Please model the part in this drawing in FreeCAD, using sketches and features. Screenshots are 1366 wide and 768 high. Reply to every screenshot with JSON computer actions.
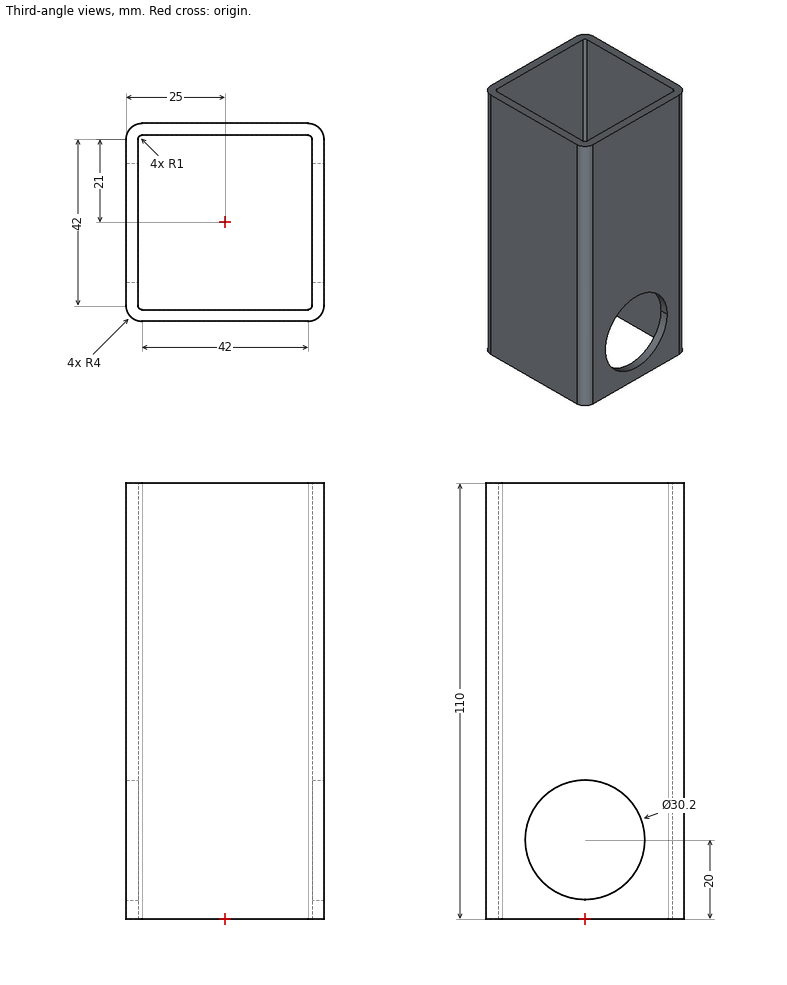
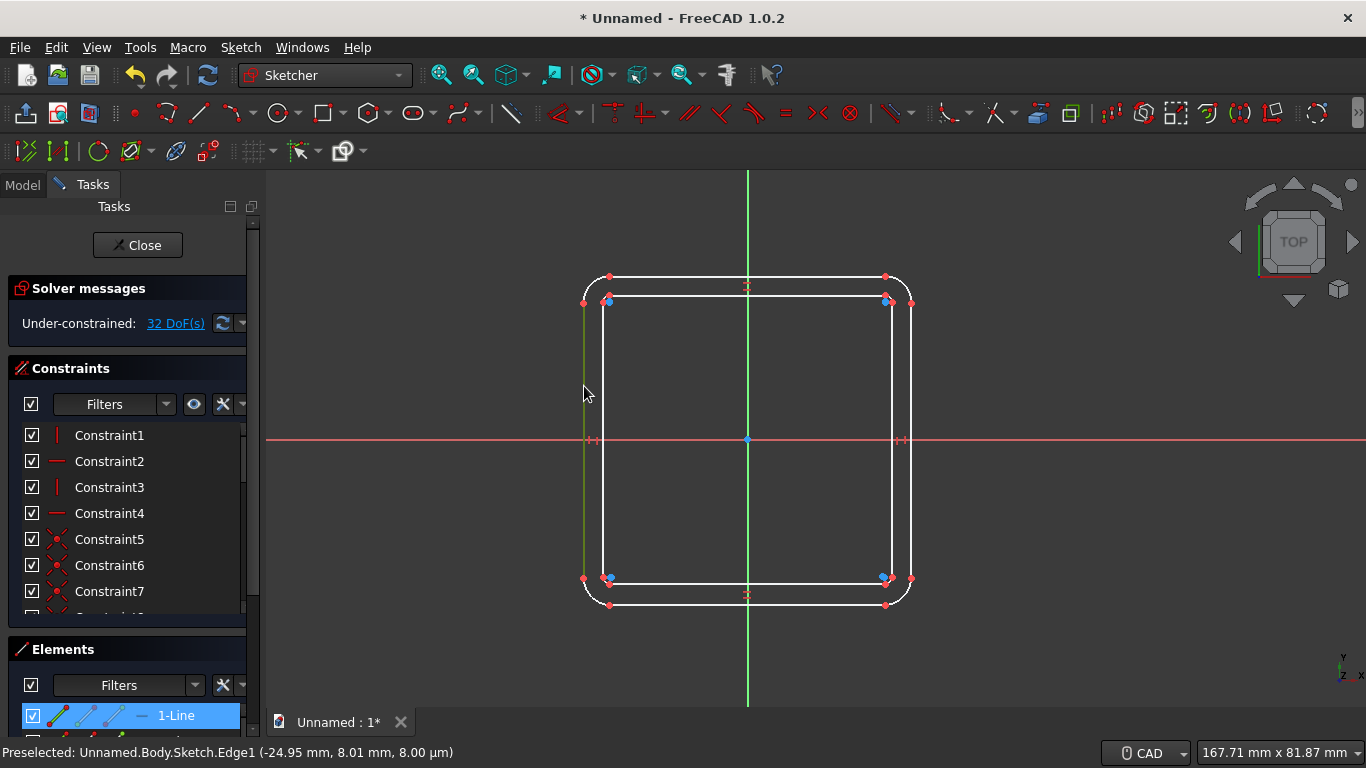
{"action": "left_click", "coordinate": [587, 590]}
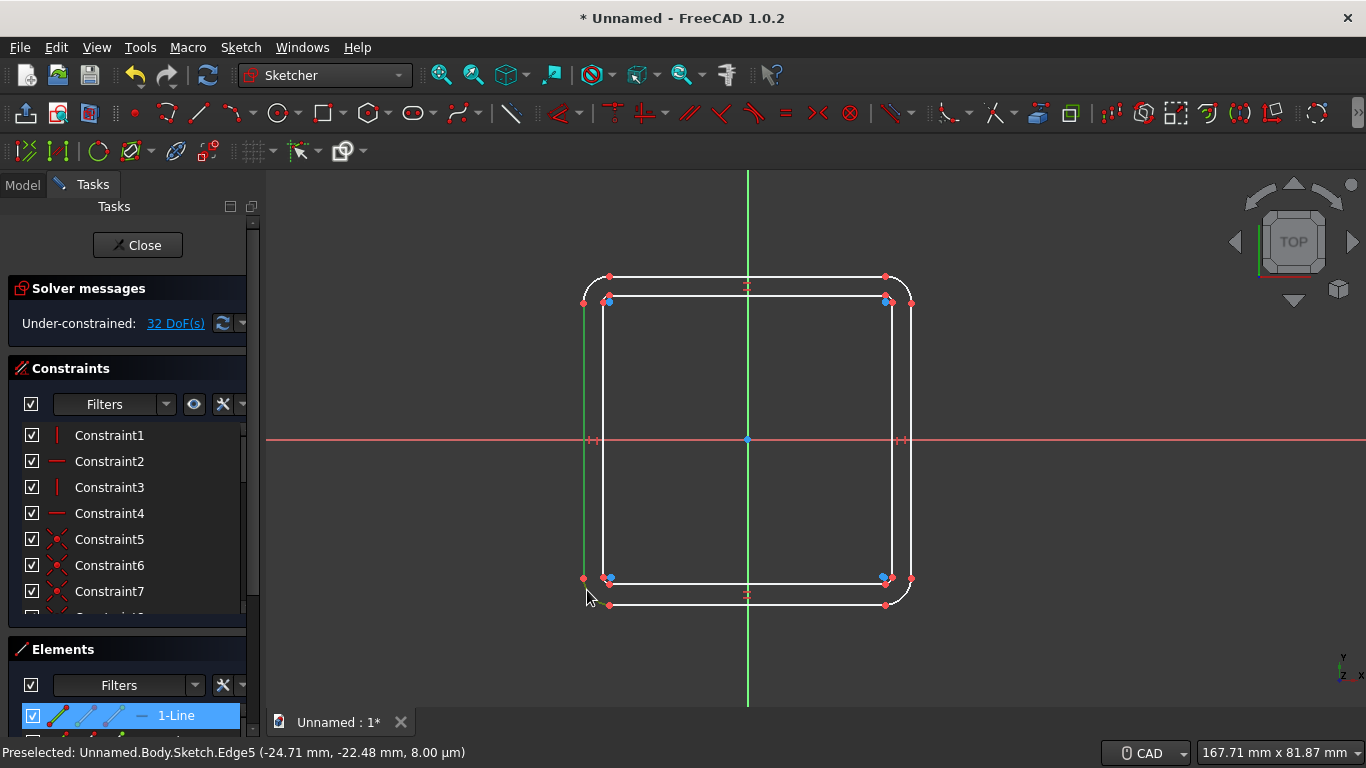
{"action": "left_click", "coordinate": [754, 114]}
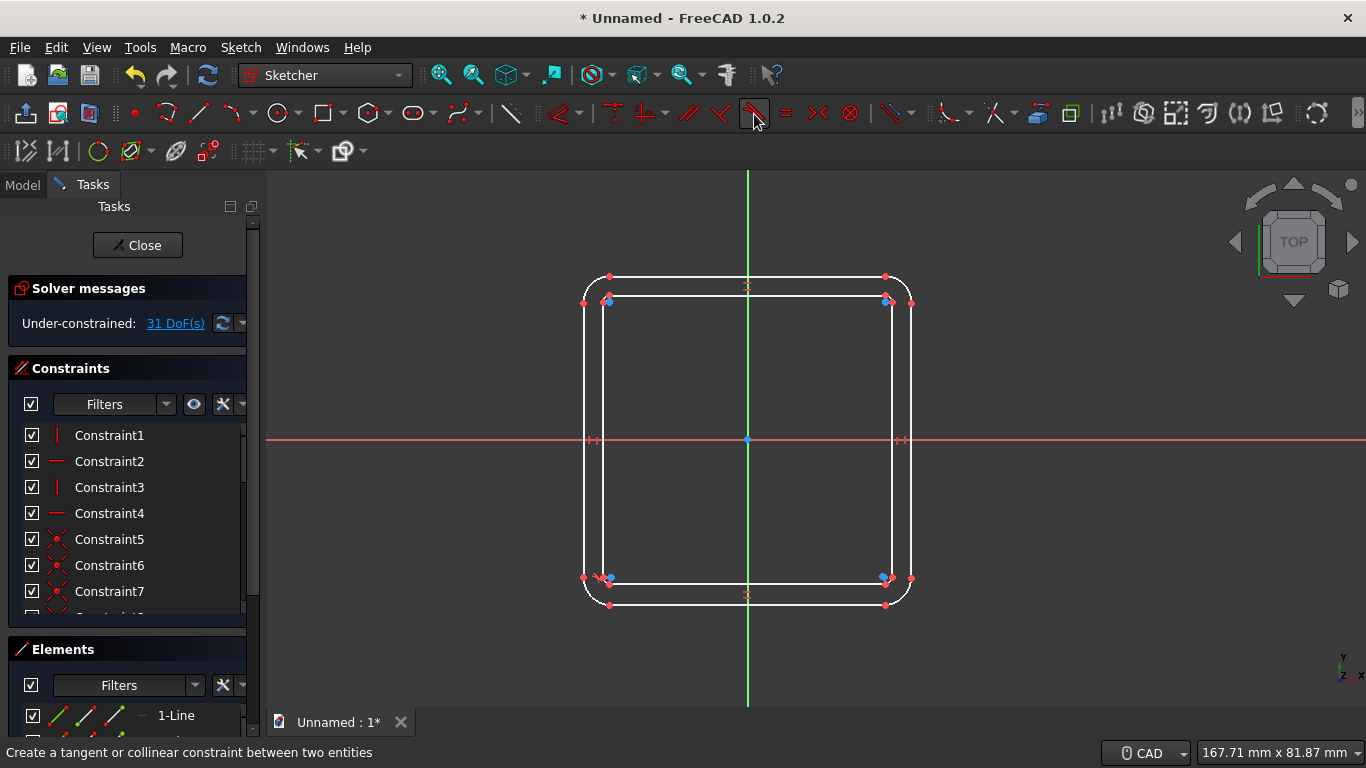
{"action": "left_click", "coordinate": [584, 386]}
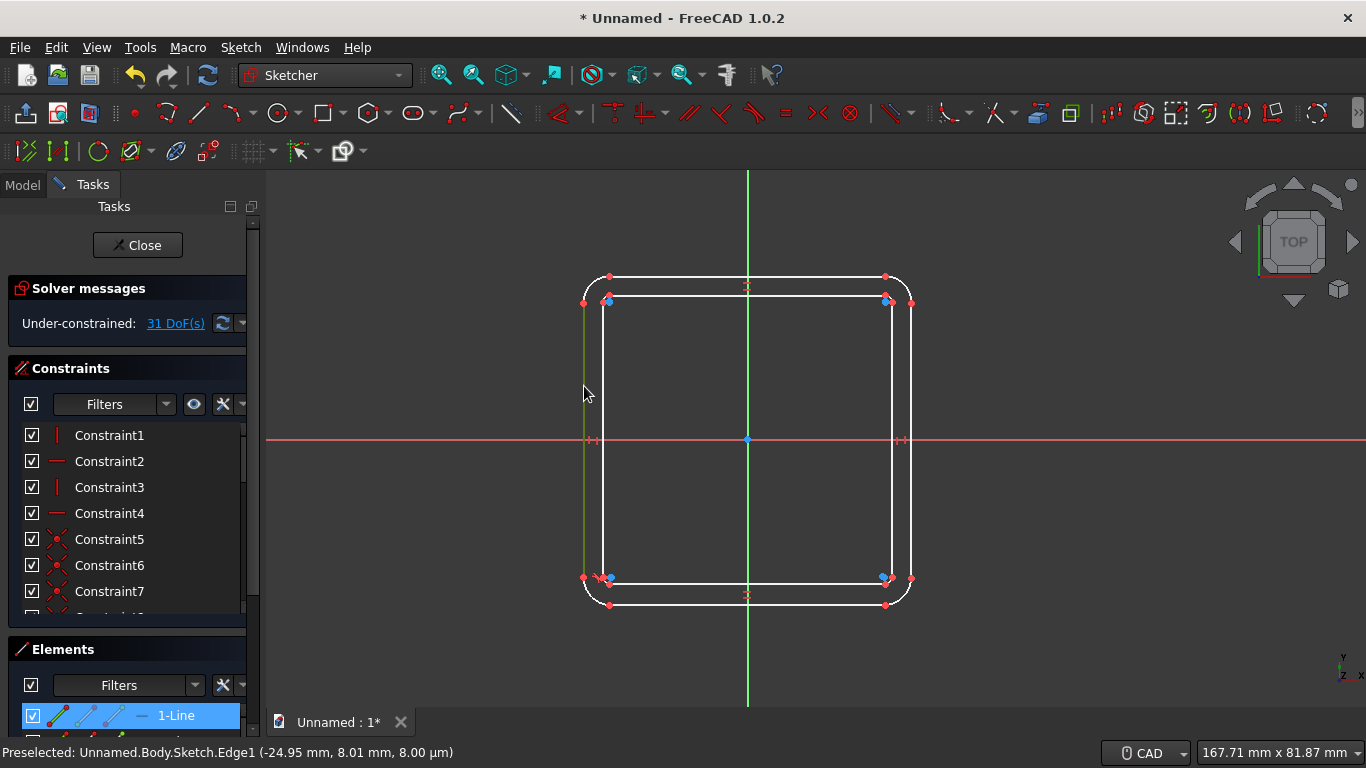
{"action": "left_click", "coordinate": [598, 279]}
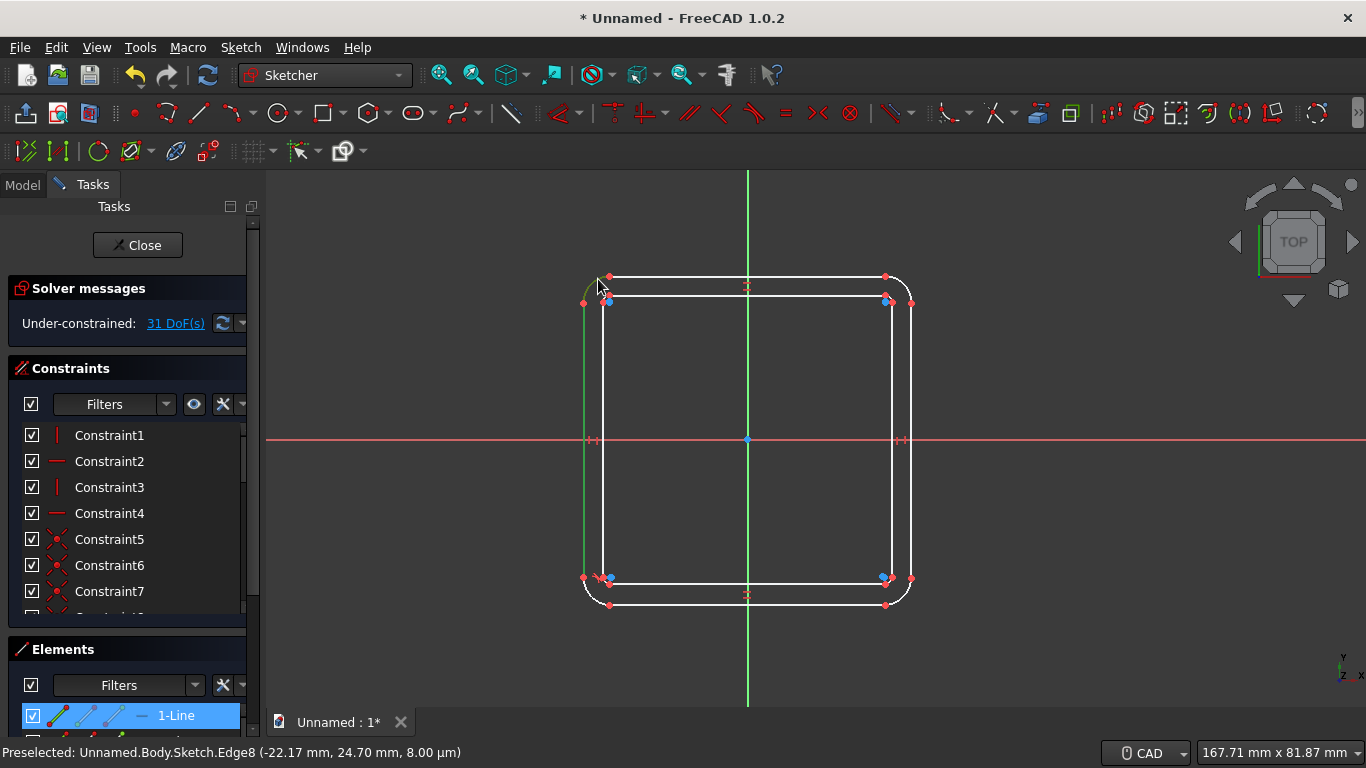
{"action": "left_click", "coordinate": [754, 114]}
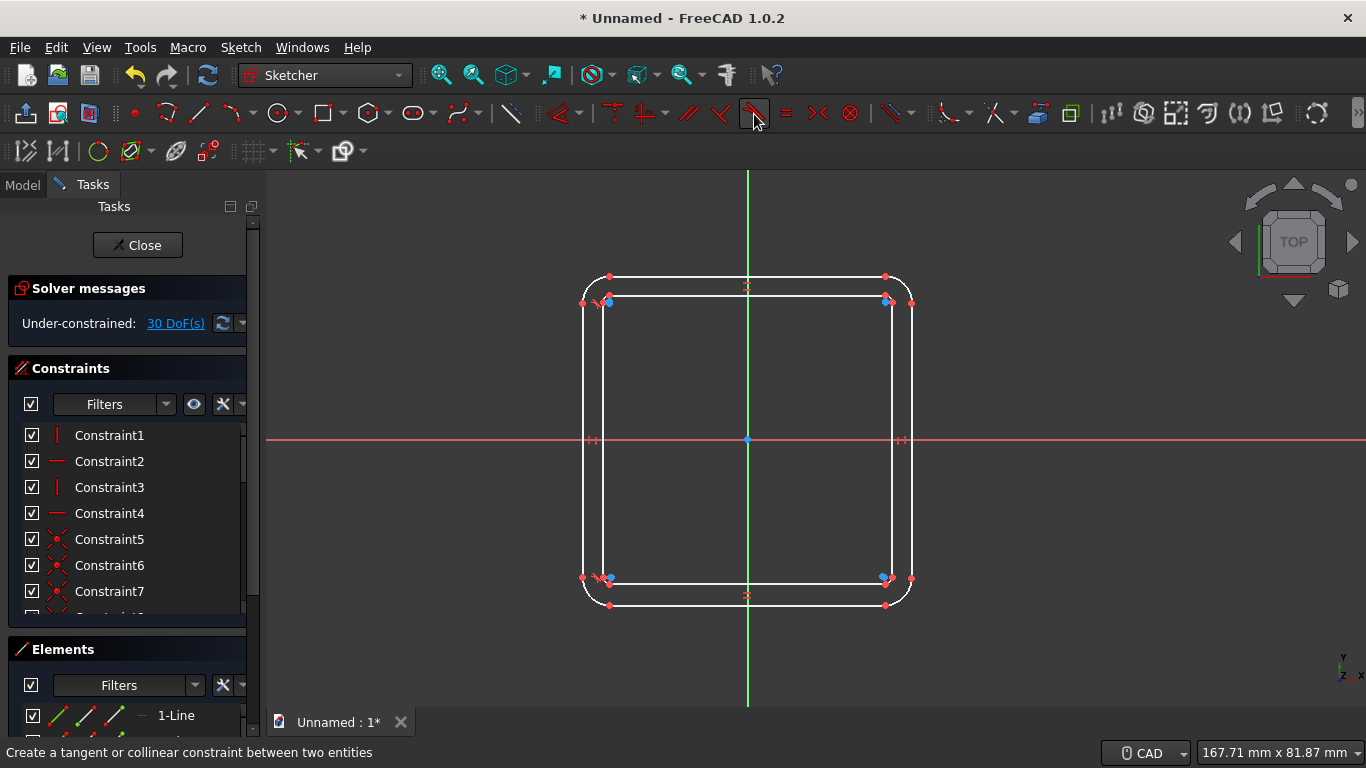
{"action": "left_click", "coordinate": [692, 606]}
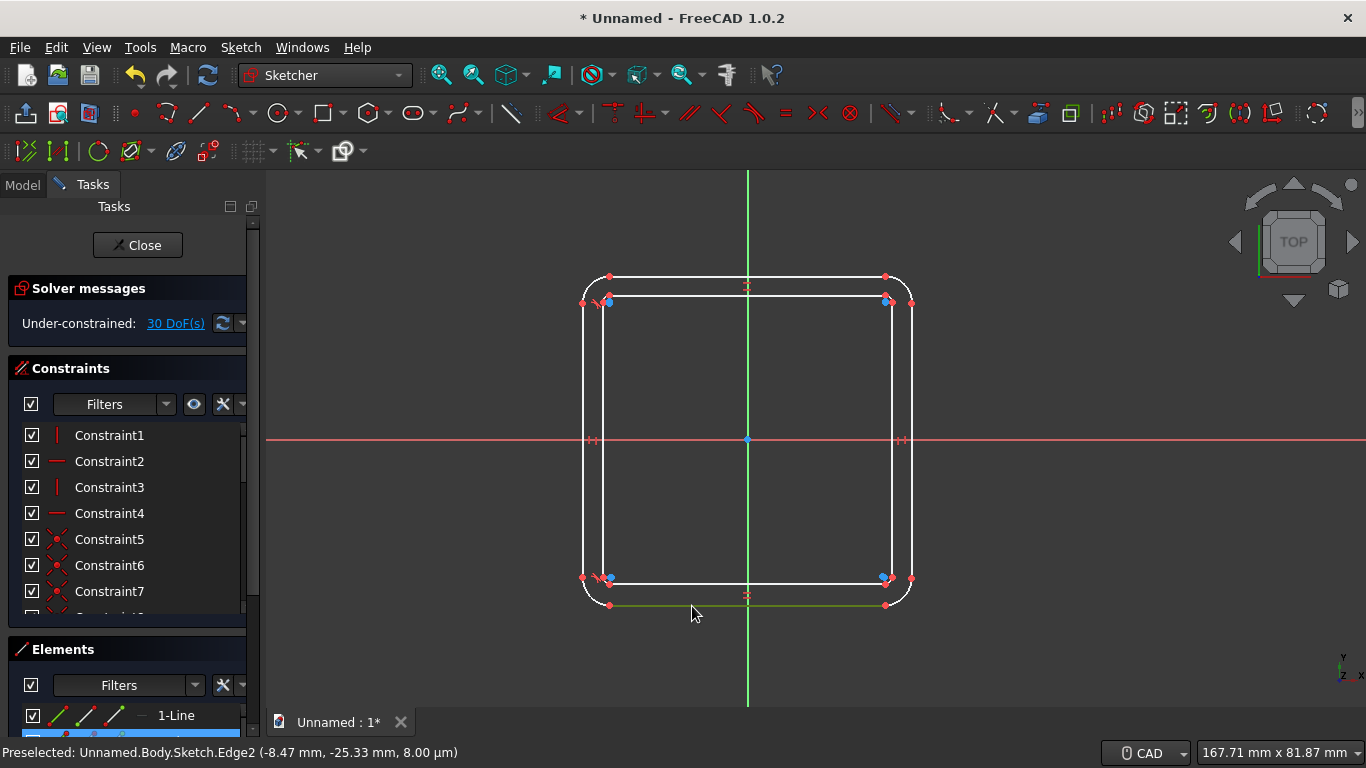
{"action": "left_click", "coordinate": [586, 590]}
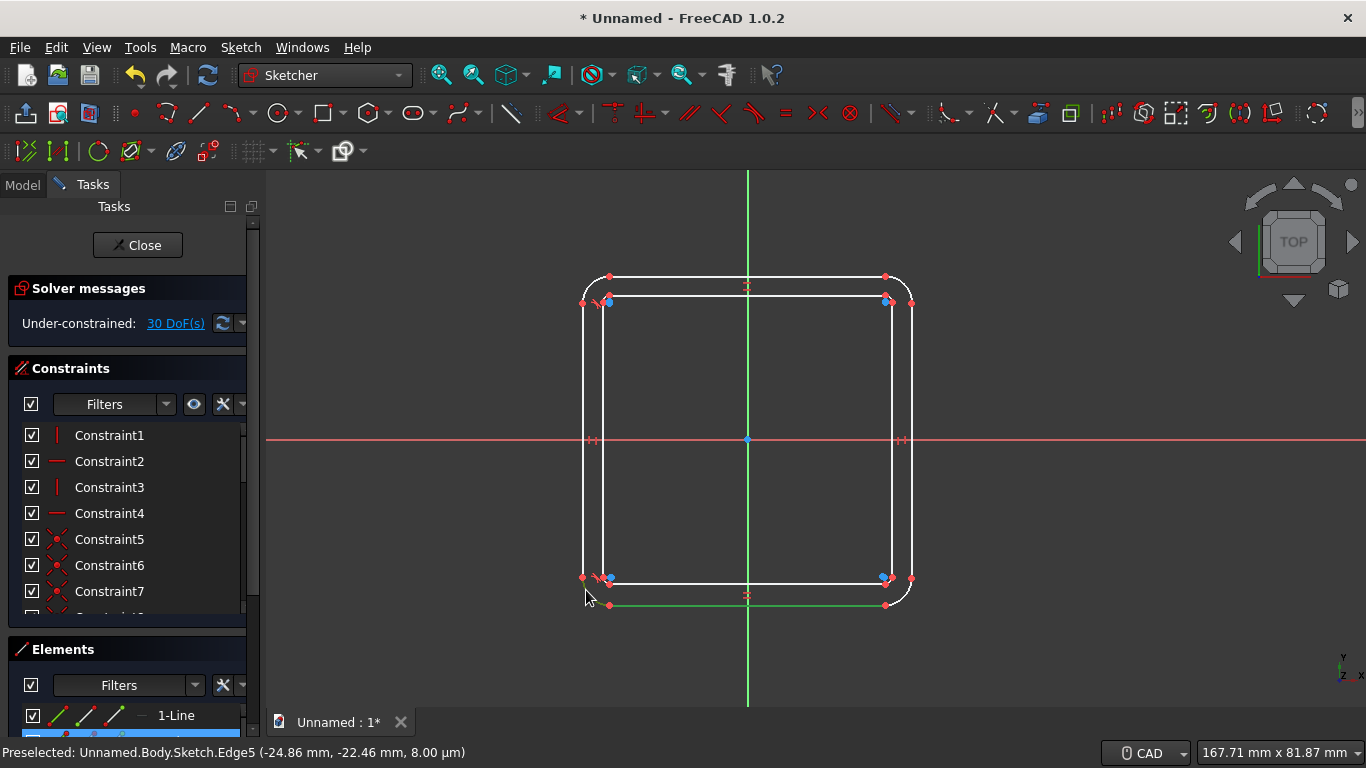
{"action": "left_click", "coordinate": [754, 114]}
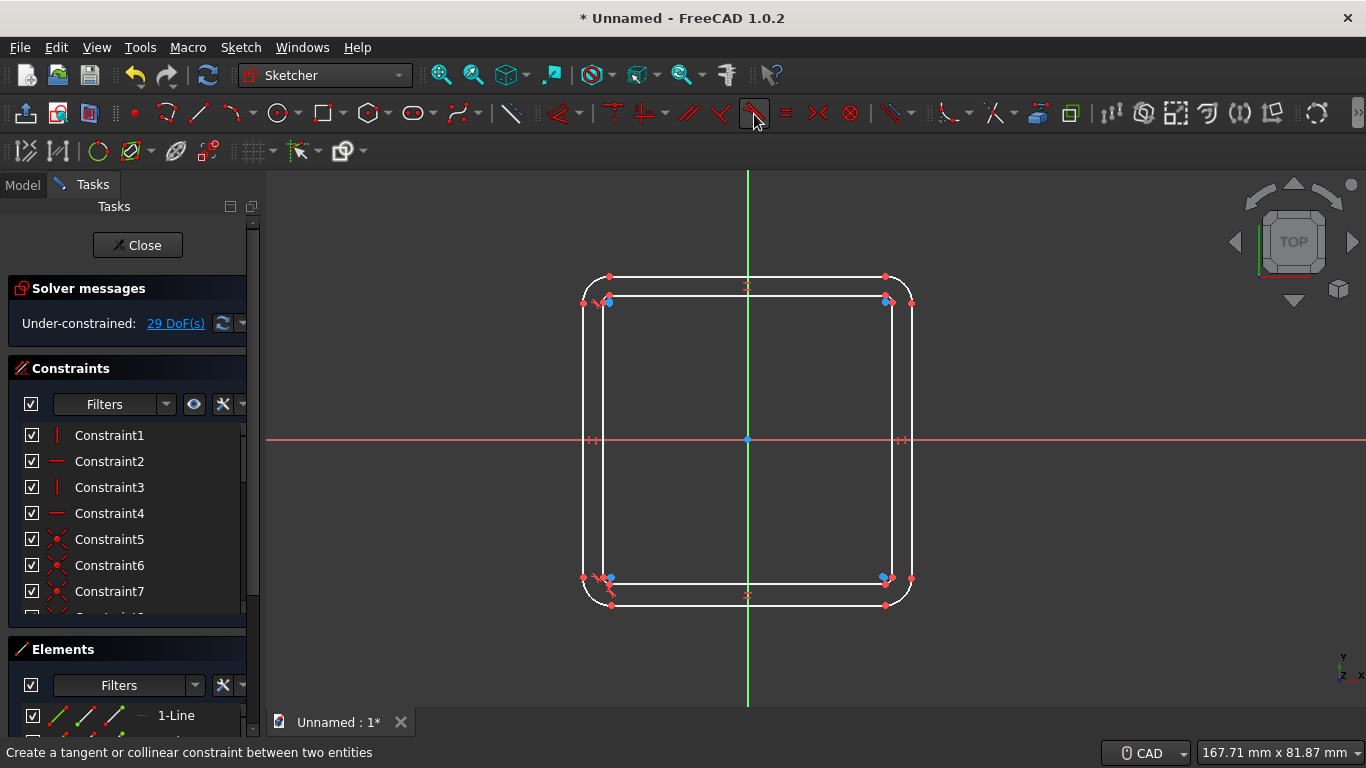
{"action": "left_click", "coordinate": [693, 606]}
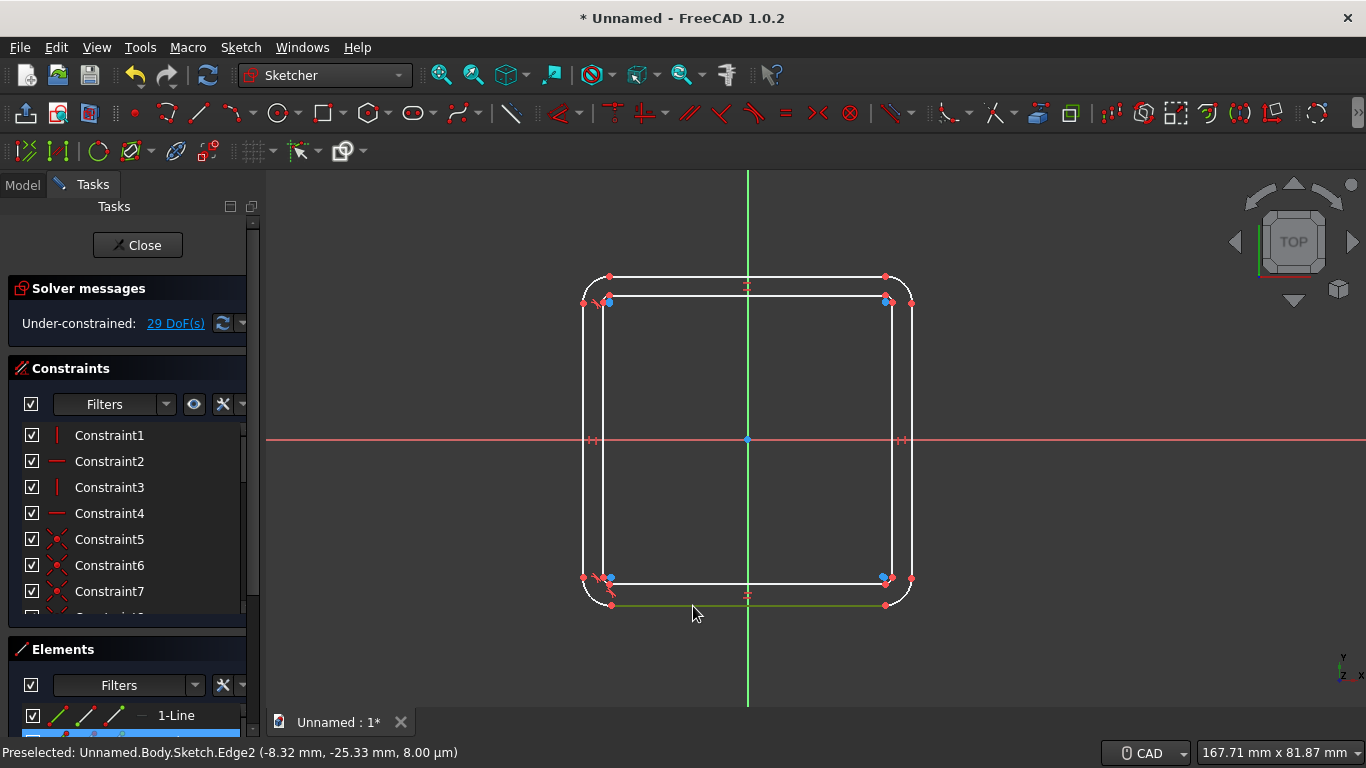
{"action": "left_click", "coordinate": [897, 602]}